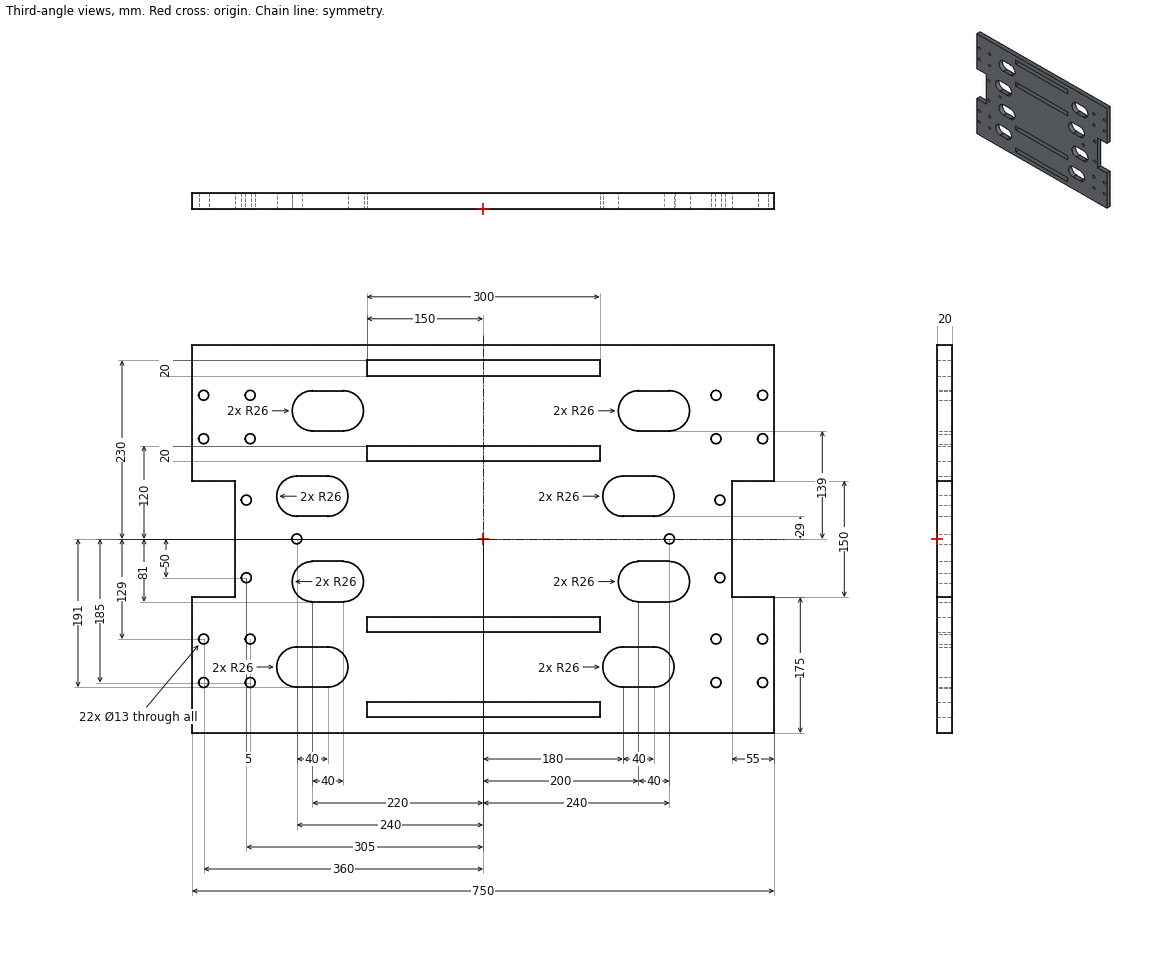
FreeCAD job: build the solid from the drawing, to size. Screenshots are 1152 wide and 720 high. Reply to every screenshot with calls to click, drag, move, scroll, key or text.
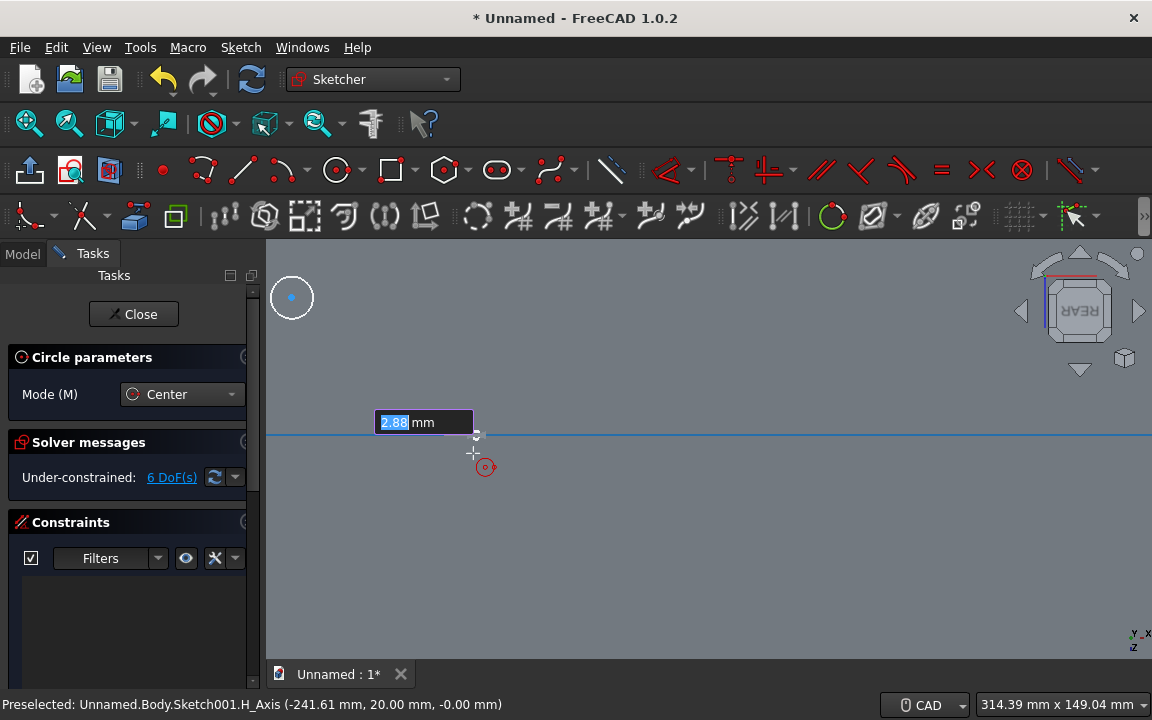
click(471, 452)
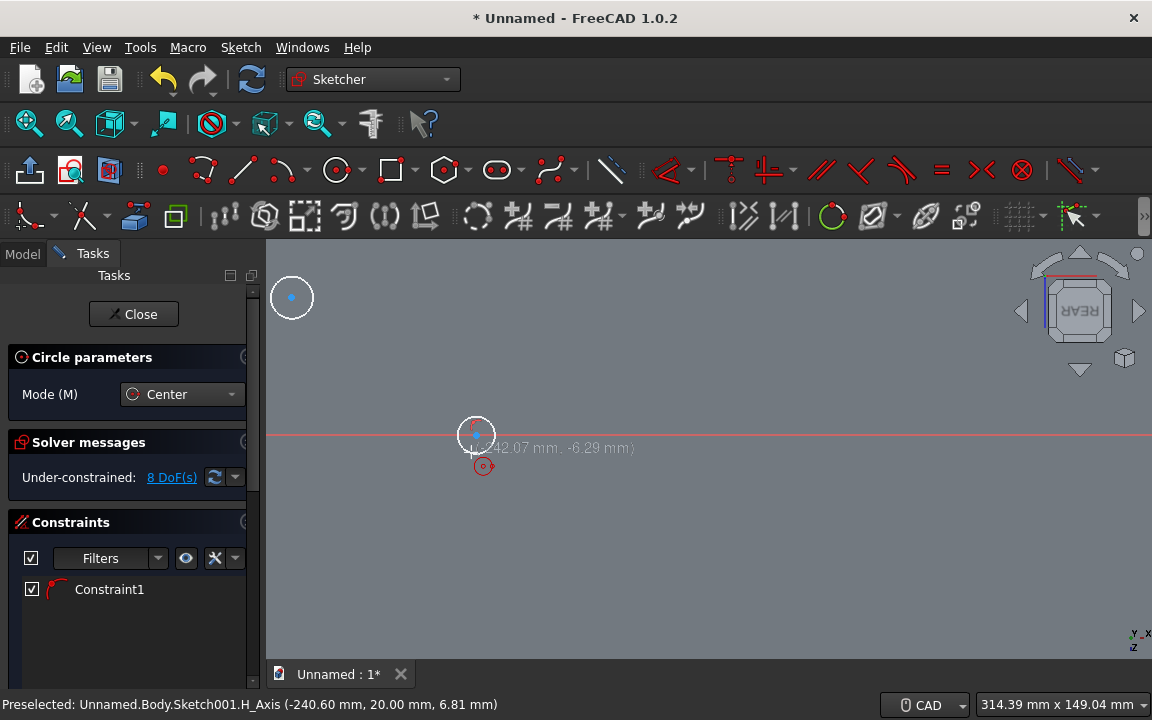
scroll(473, 453, down, 7)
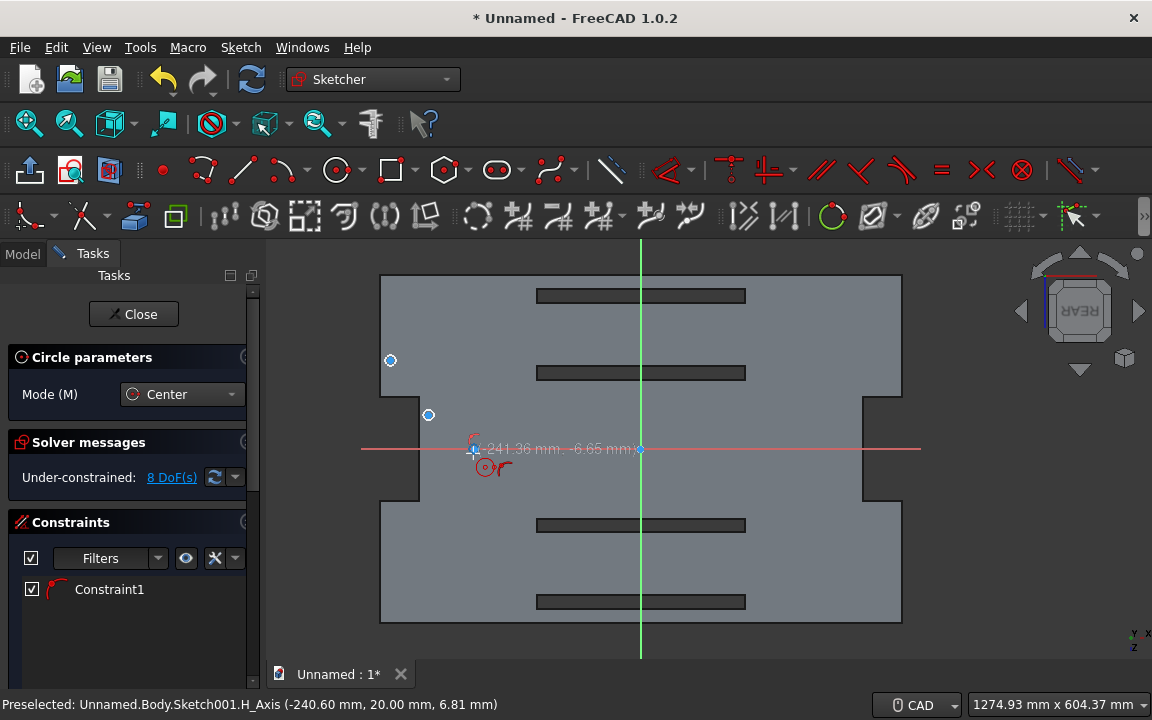
scroll(432, 359, up, 9)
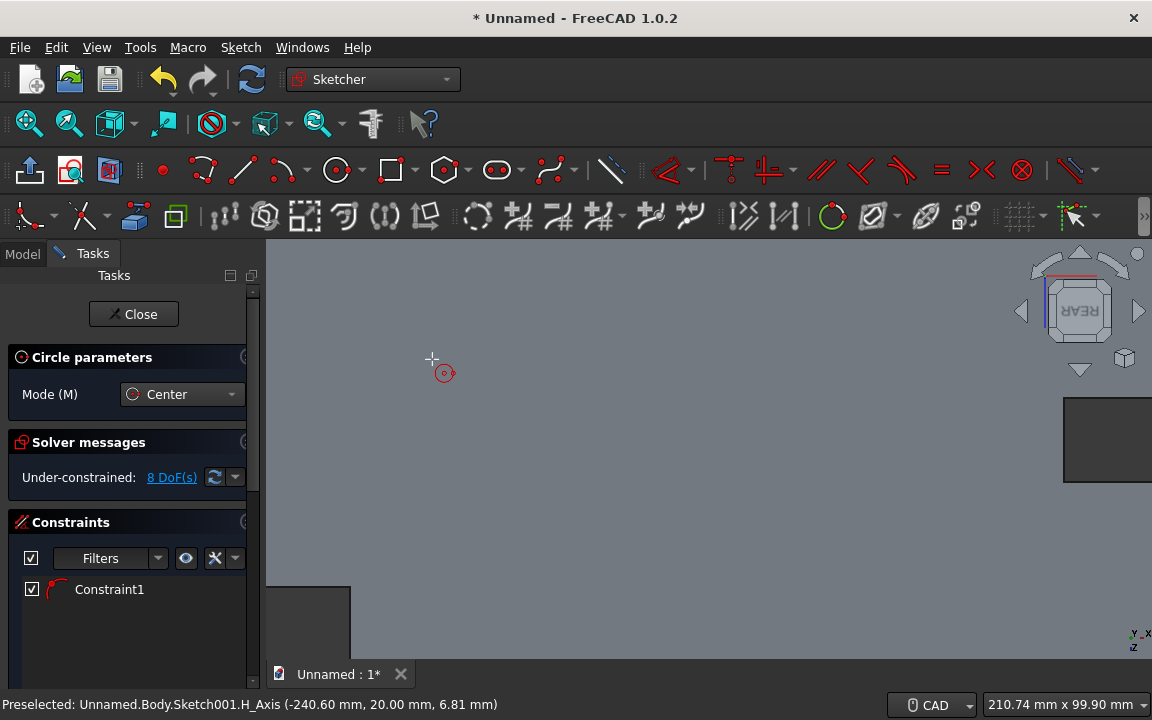
scroll(432, 359, down, 9)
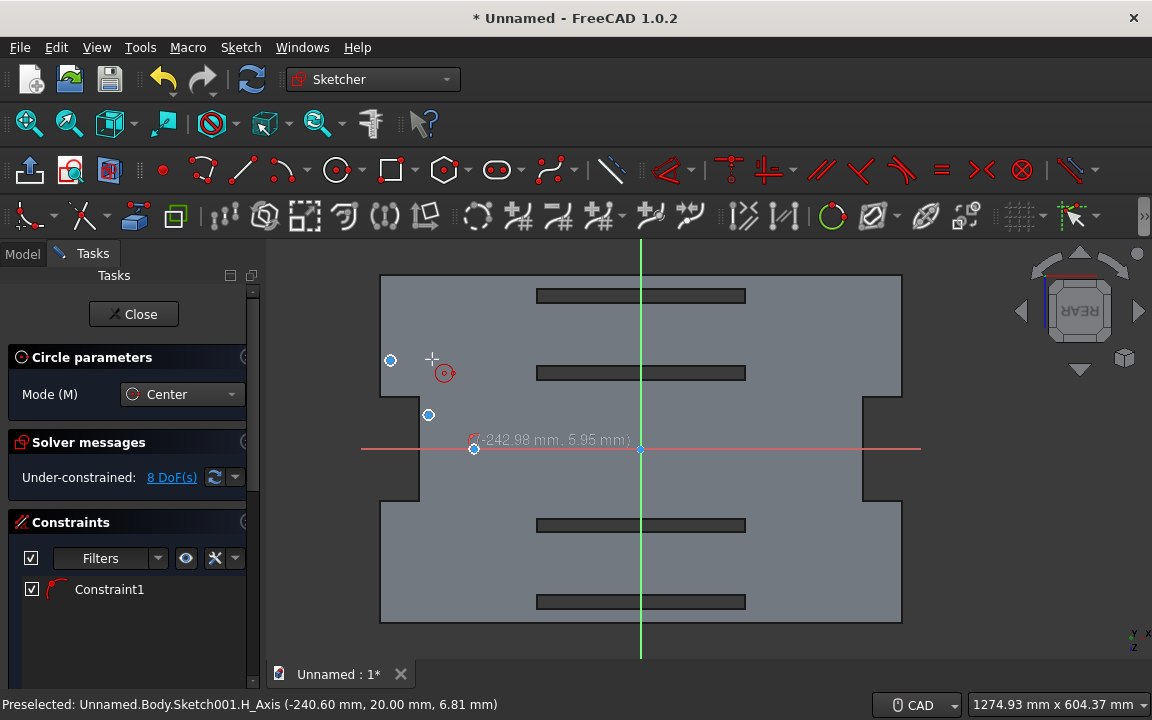
click(432, 359)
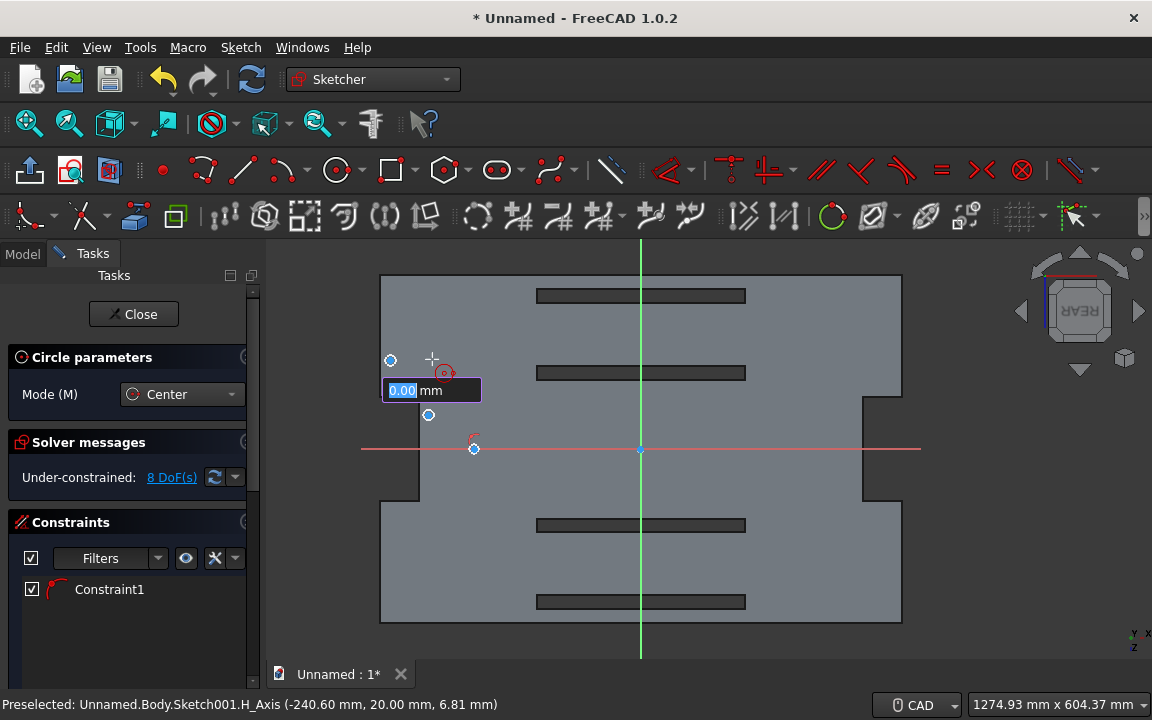
scroll(436, 356, up, 7)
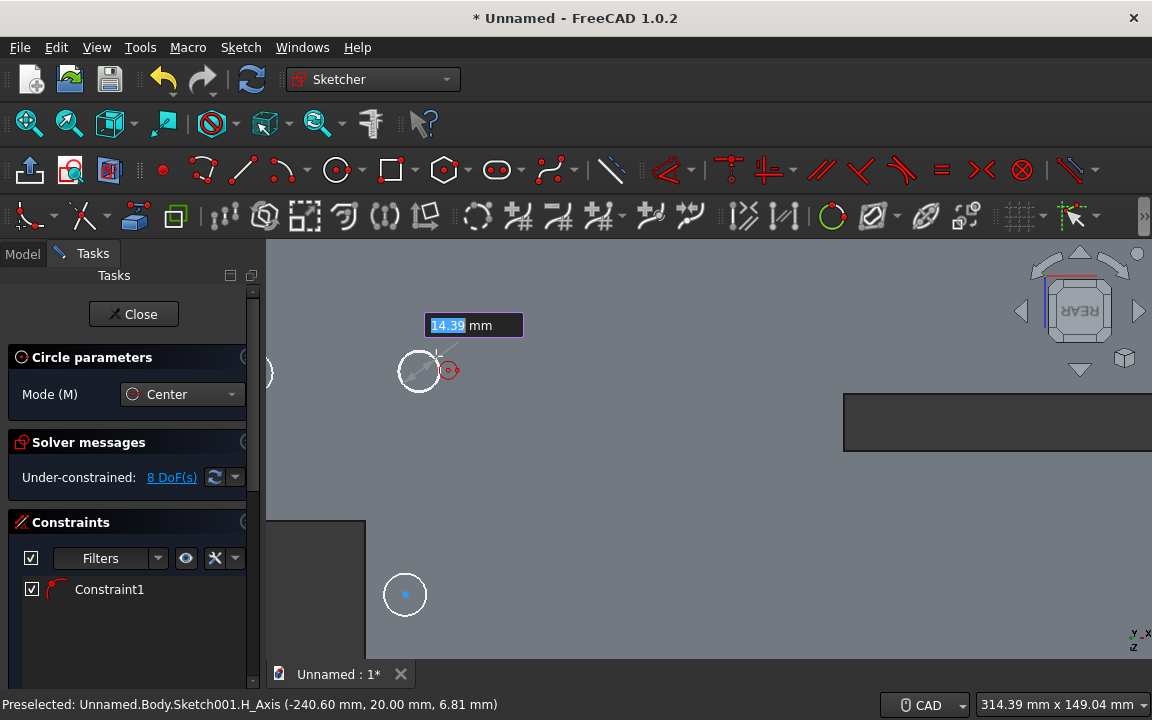
click(434, 356)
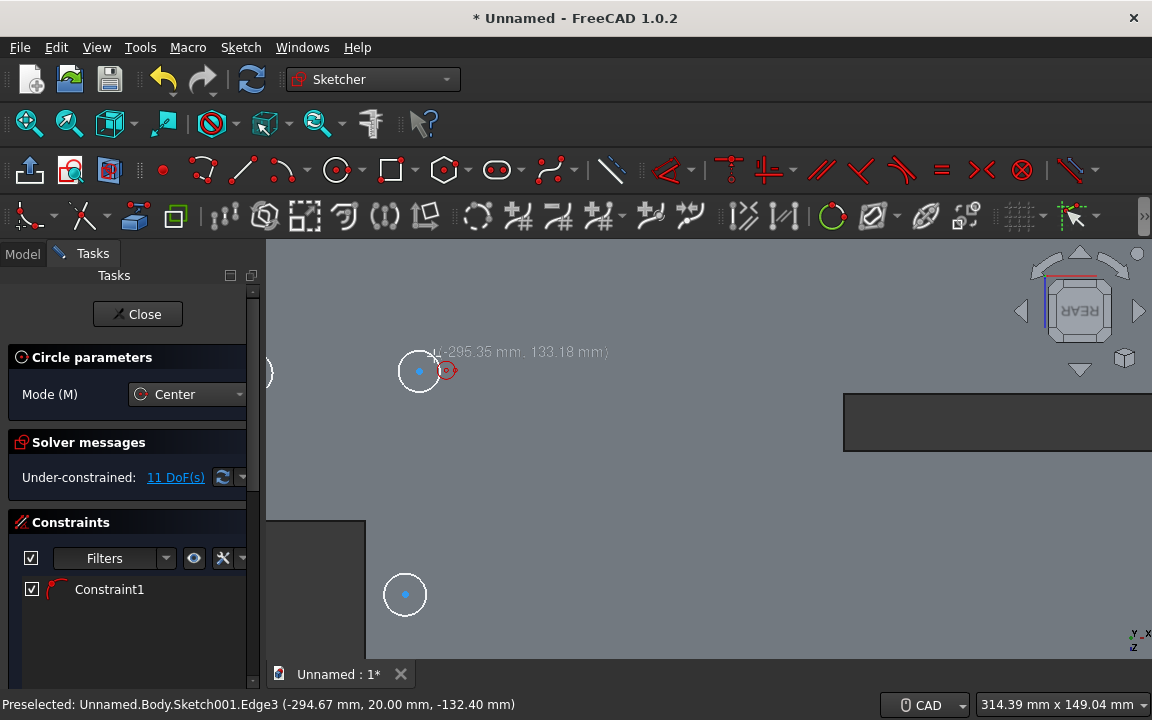
scroll(436, 356, down, 7)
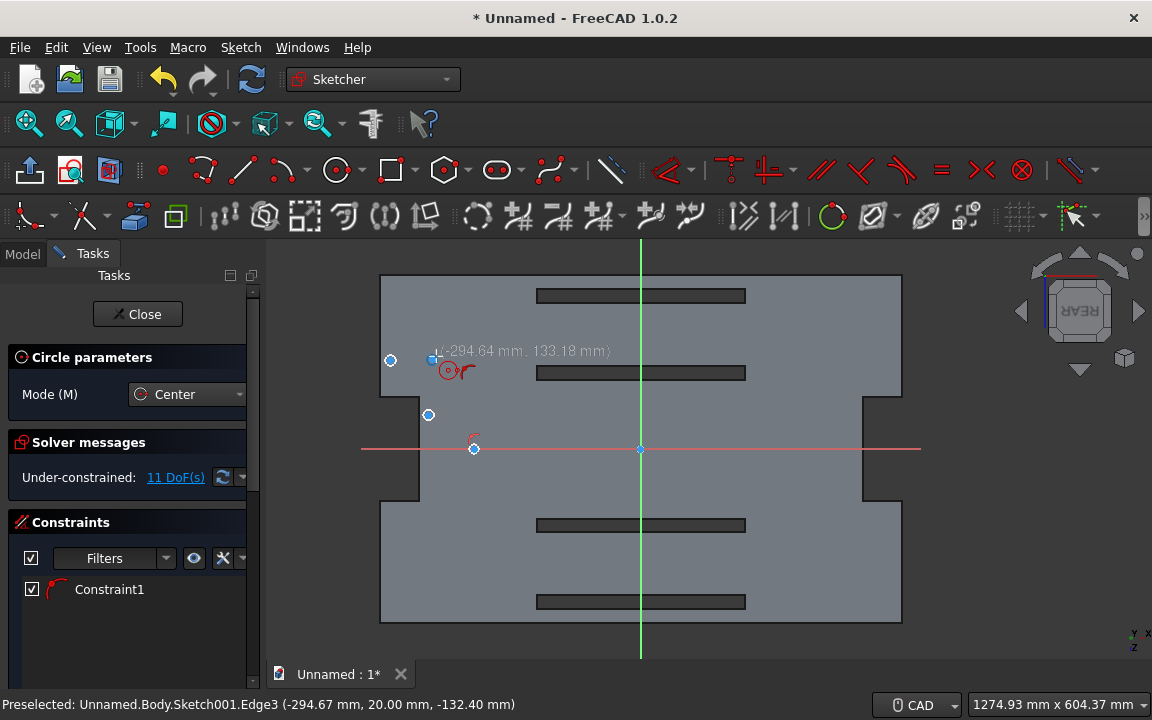
scroll(432, 320, up, 9)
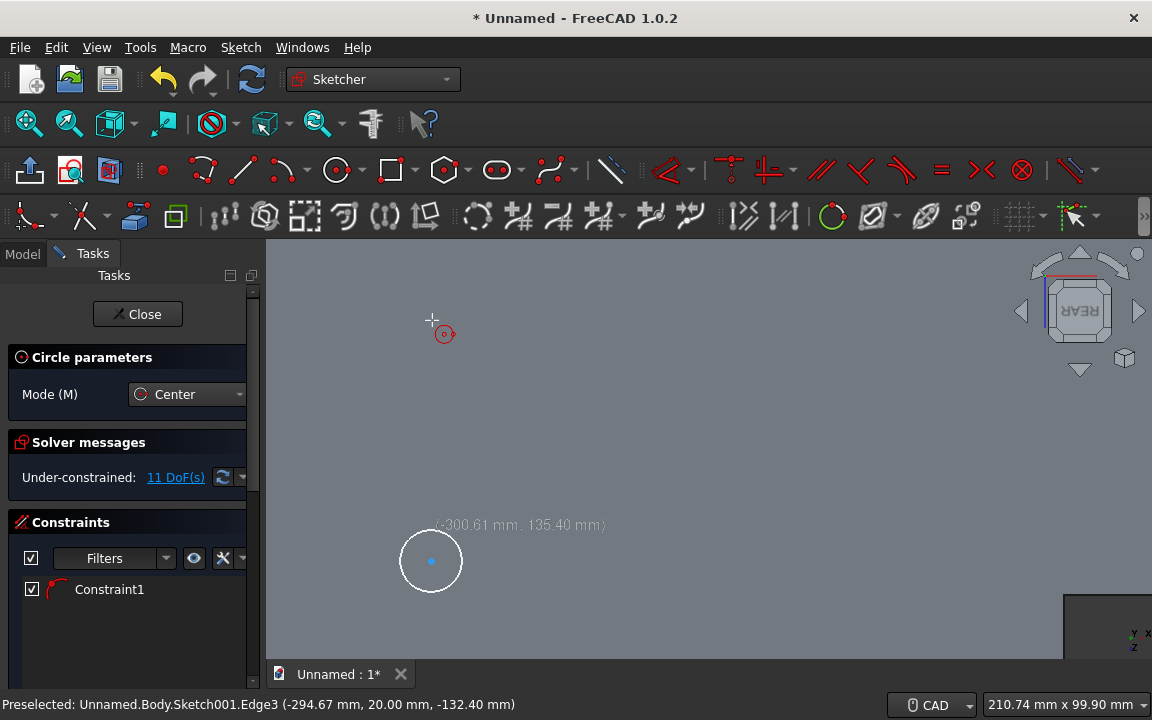
scroll(432, 320, down, 9)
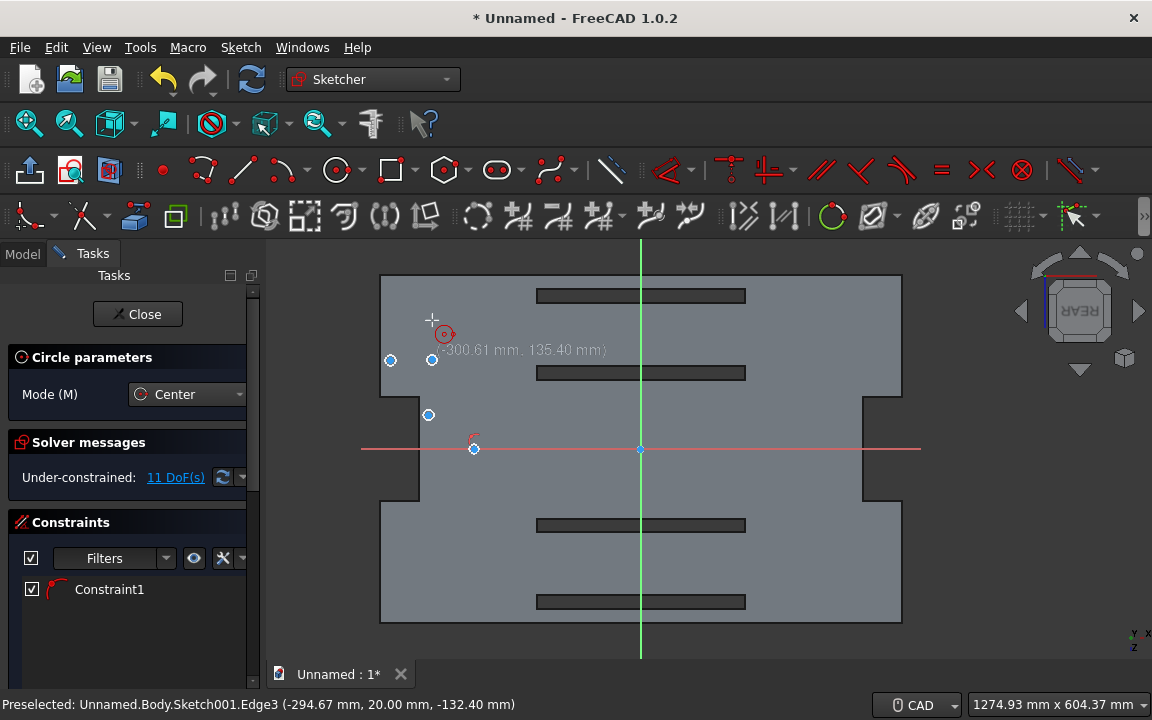
click(432, 320)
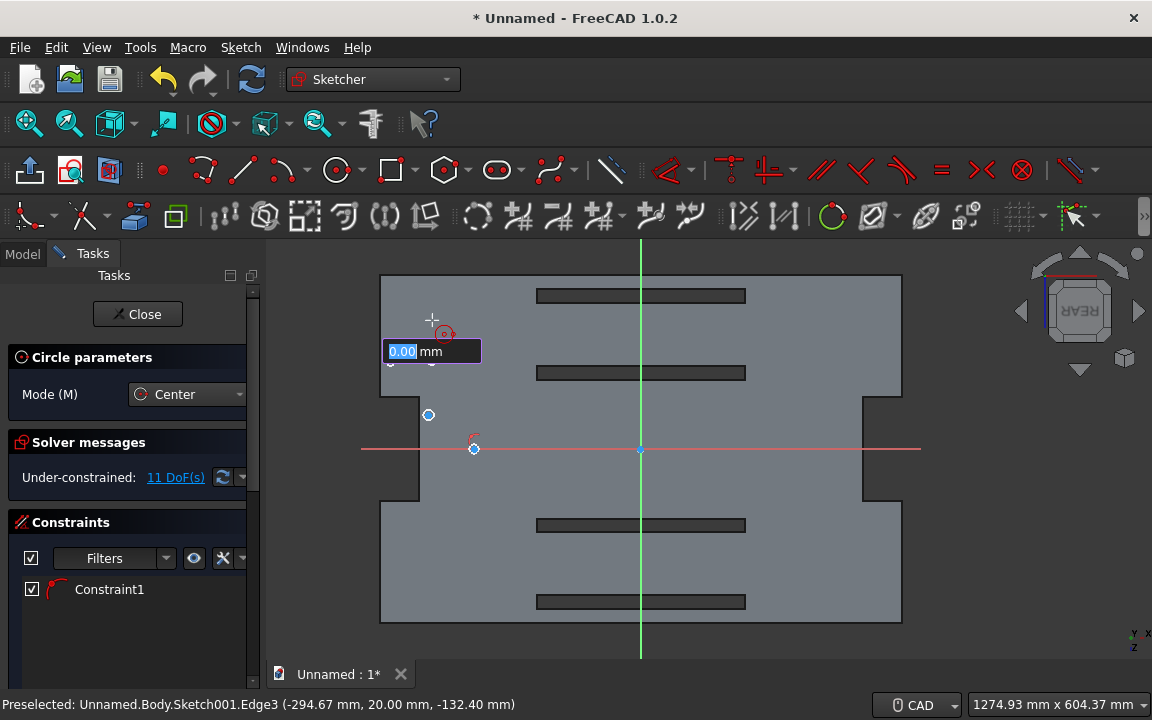
scroll(436, 317, up, 7)